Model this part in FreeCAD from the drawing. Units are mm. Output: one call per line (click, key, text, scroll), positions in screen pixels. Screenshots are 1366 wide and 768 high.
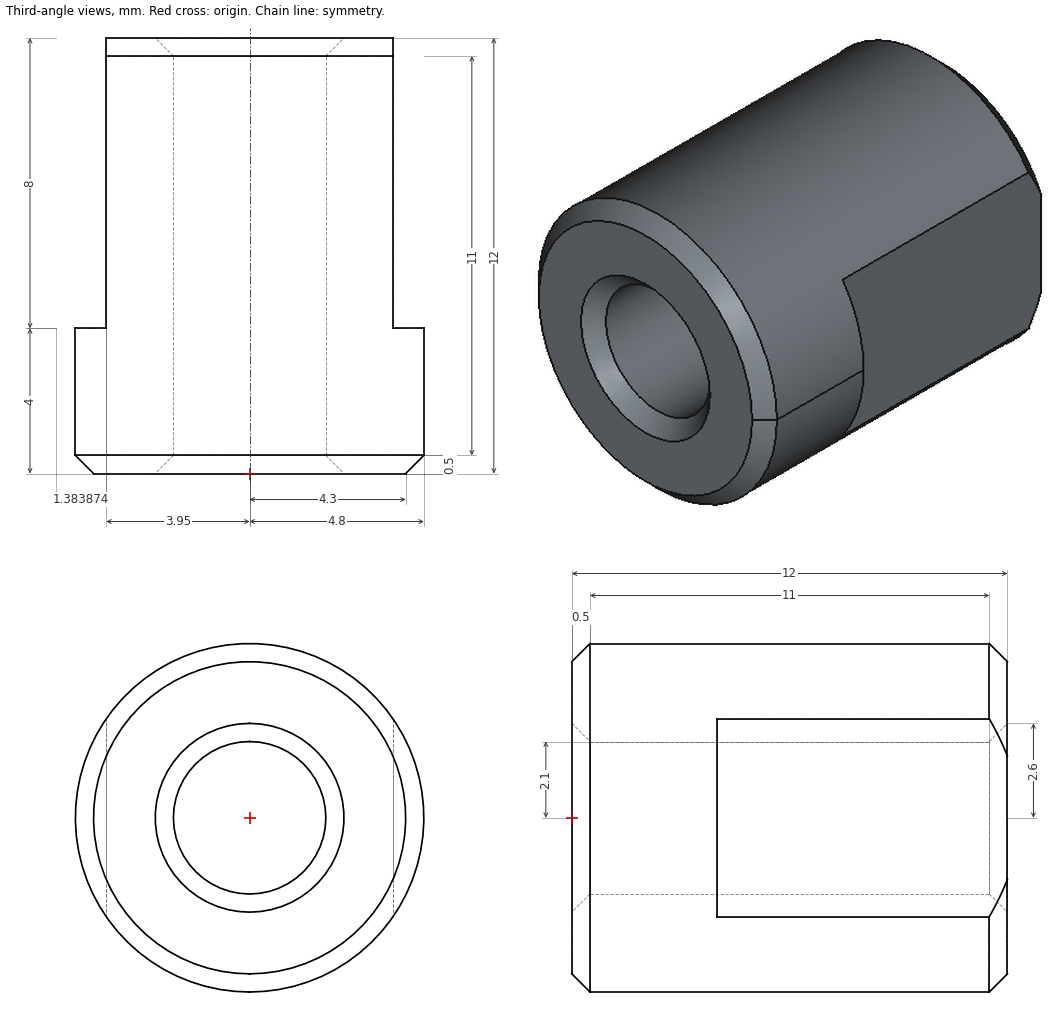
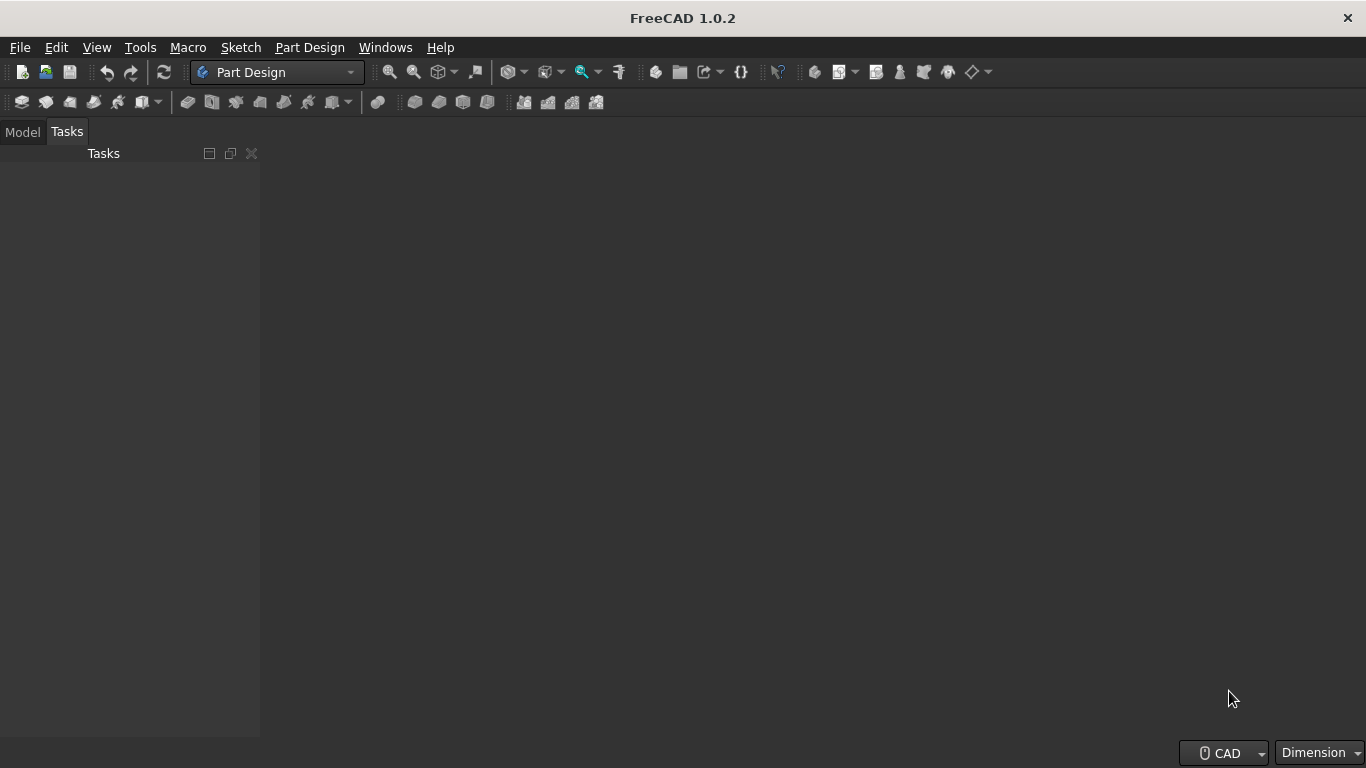
click(22, 72)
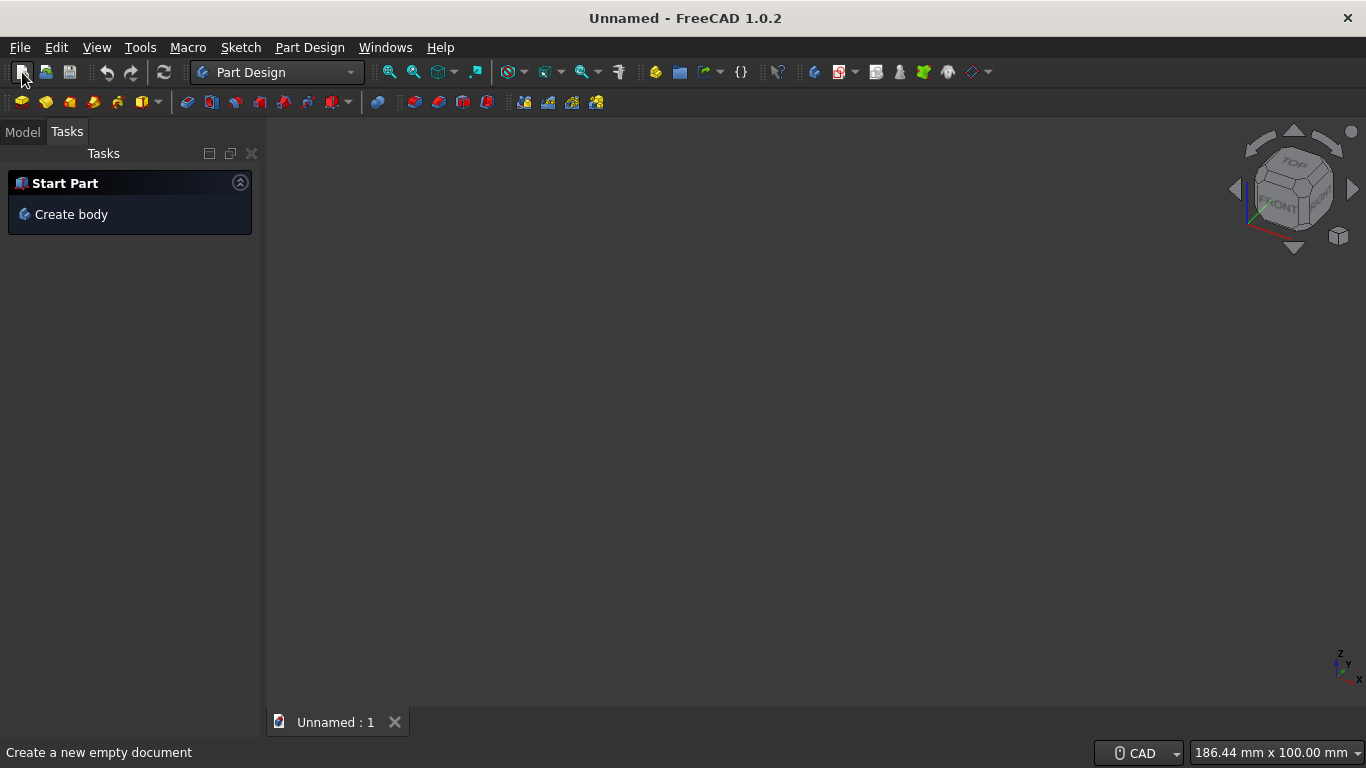
click(840, 72)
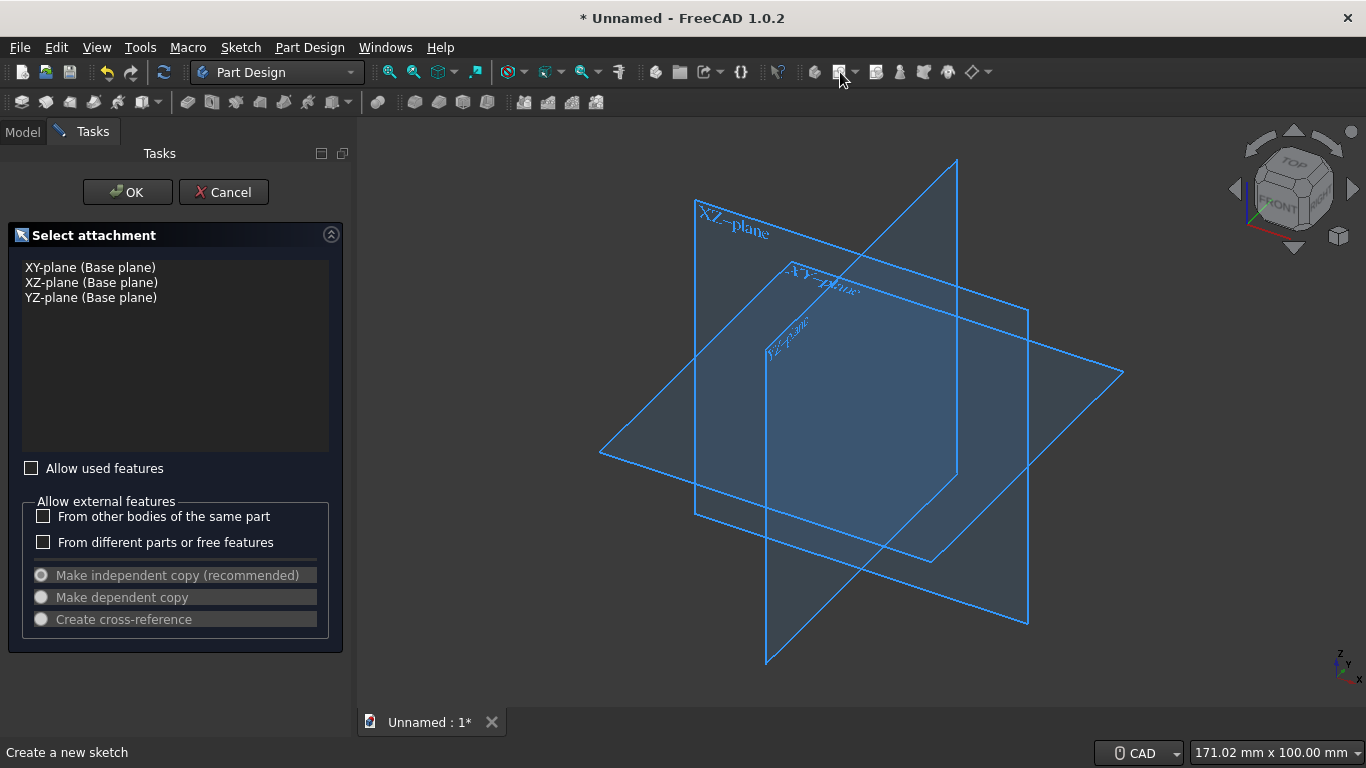
click(82, 268)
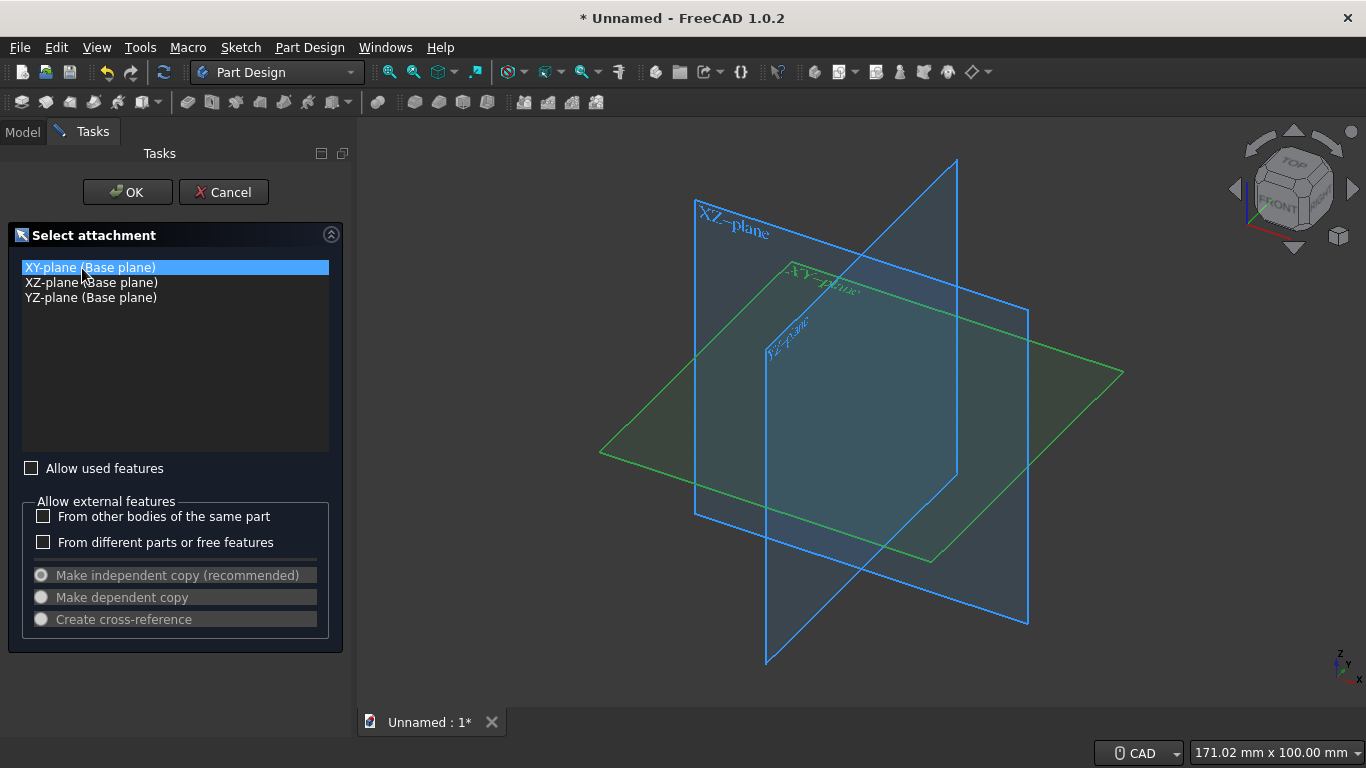
click(128, 192)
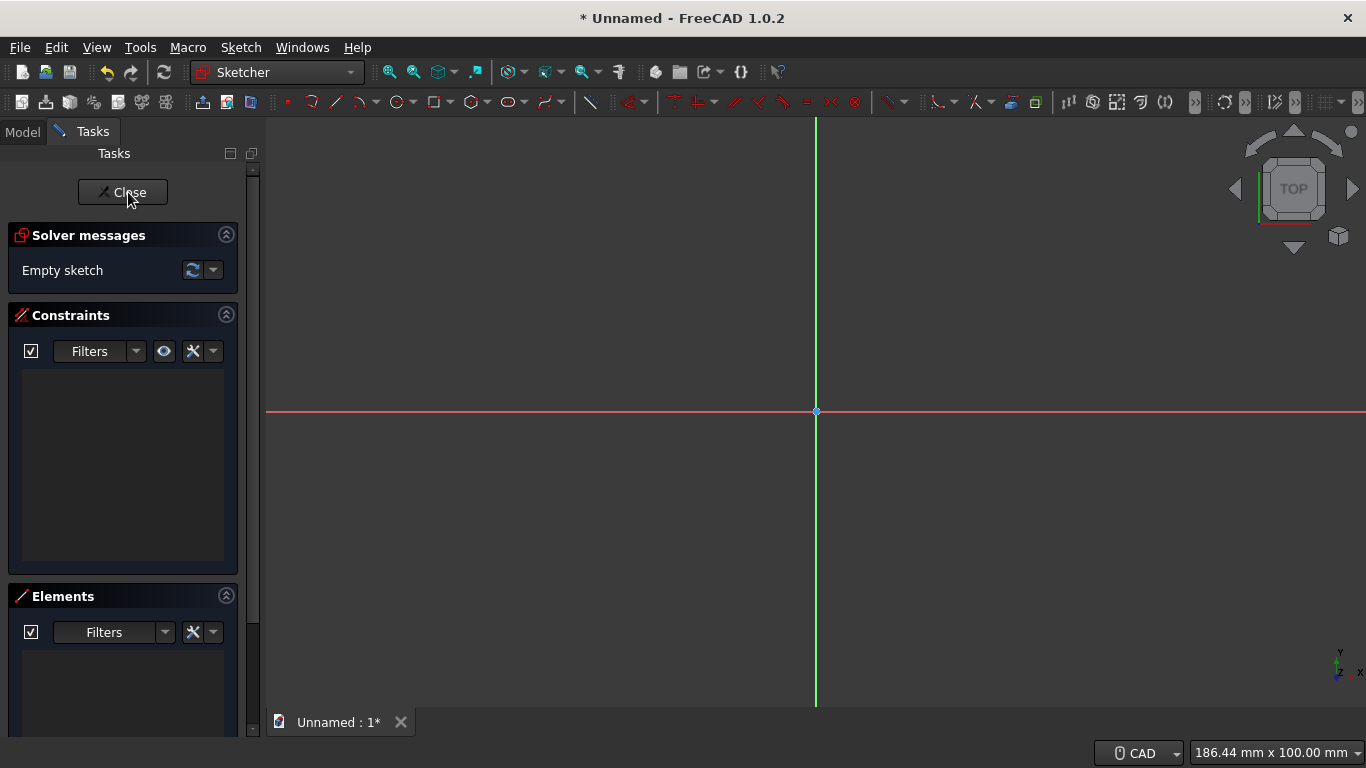
scroll(851, 368, up, 8)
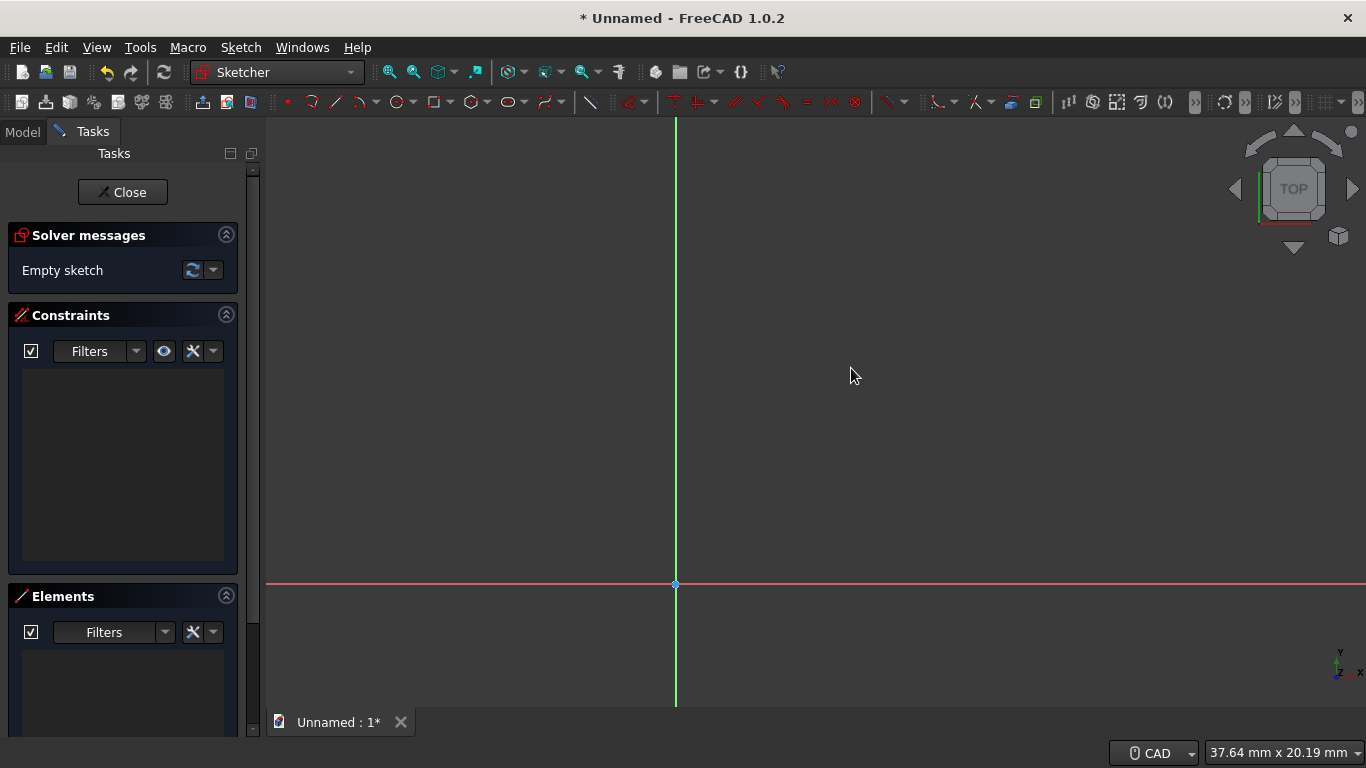
click(312, 102)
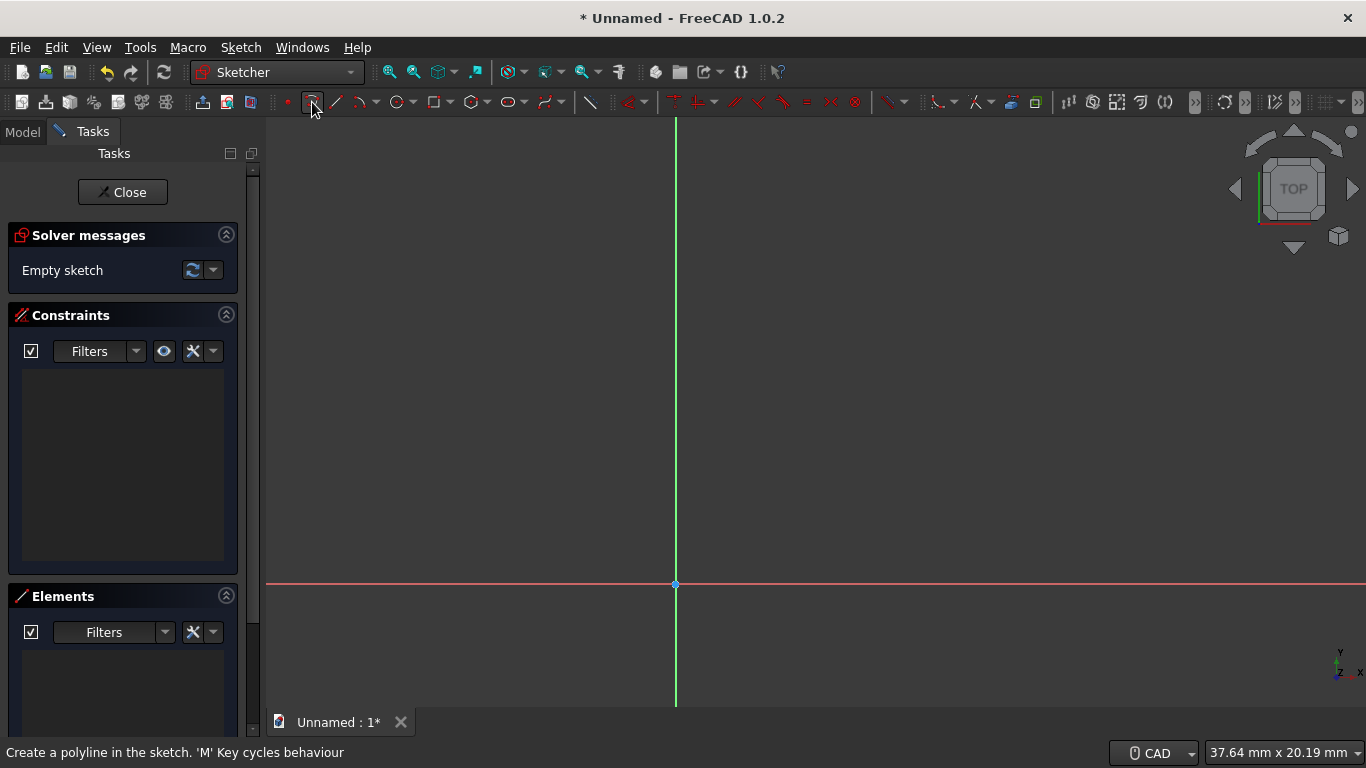
click(676, 584)
click(801, 575)
click(816, 570)
click(816, 248)
click(801, 234)
click(685, 234)
click(676, 584)
key(Escape)
key(Escape)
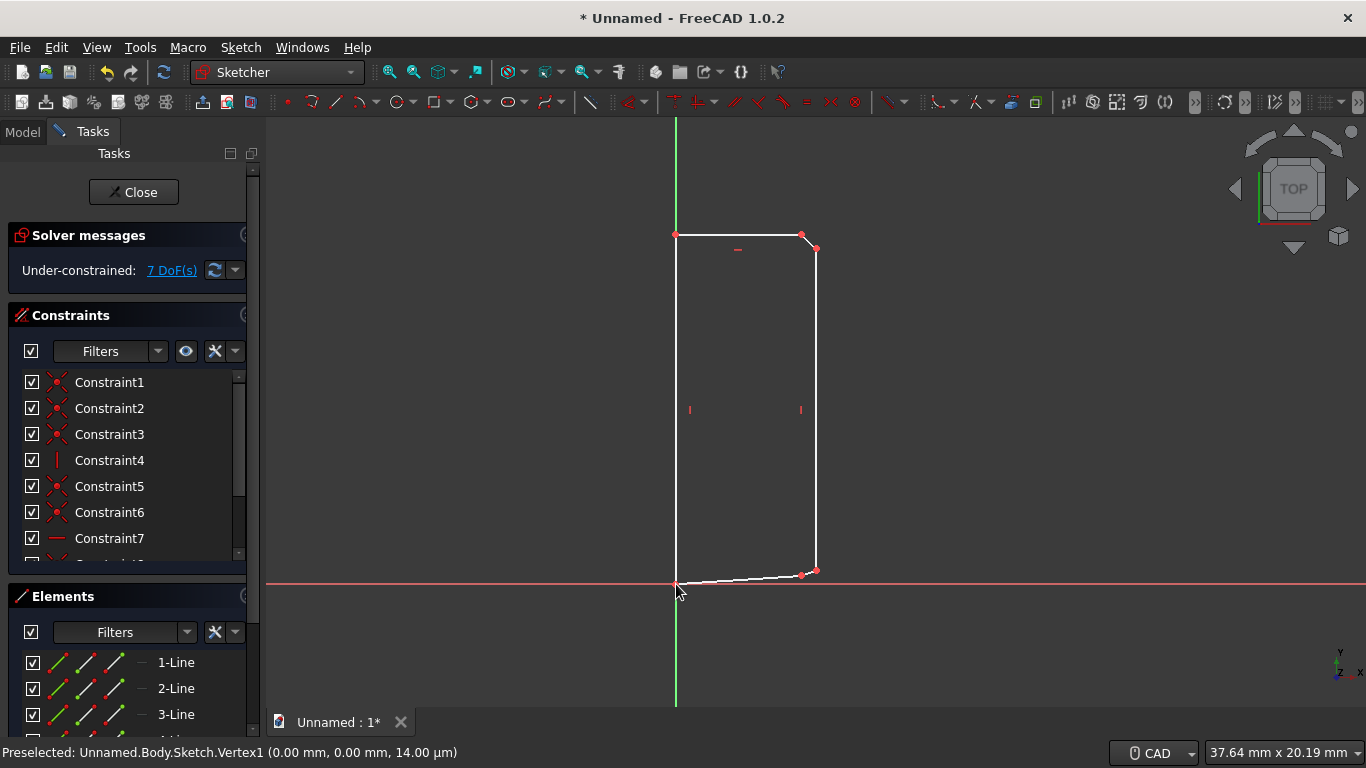
click(713, 582)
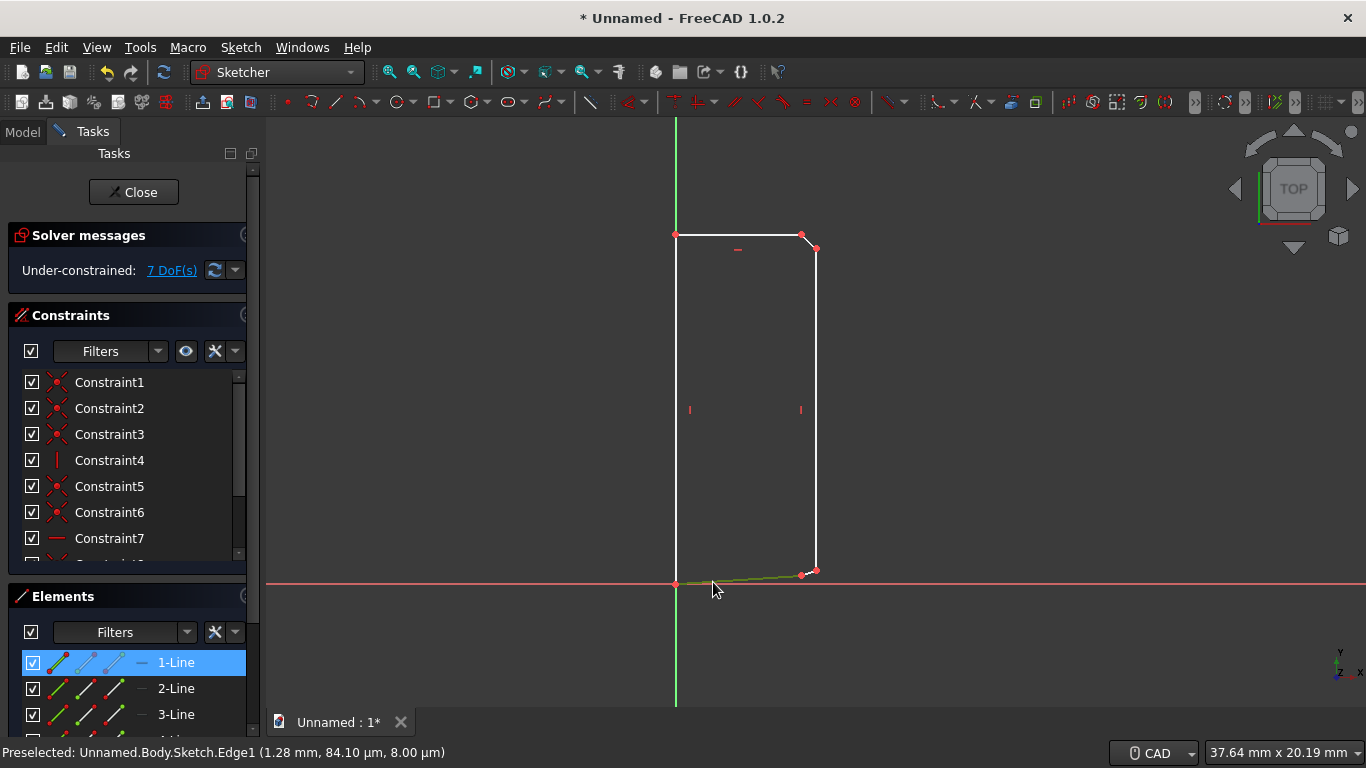
key(h)